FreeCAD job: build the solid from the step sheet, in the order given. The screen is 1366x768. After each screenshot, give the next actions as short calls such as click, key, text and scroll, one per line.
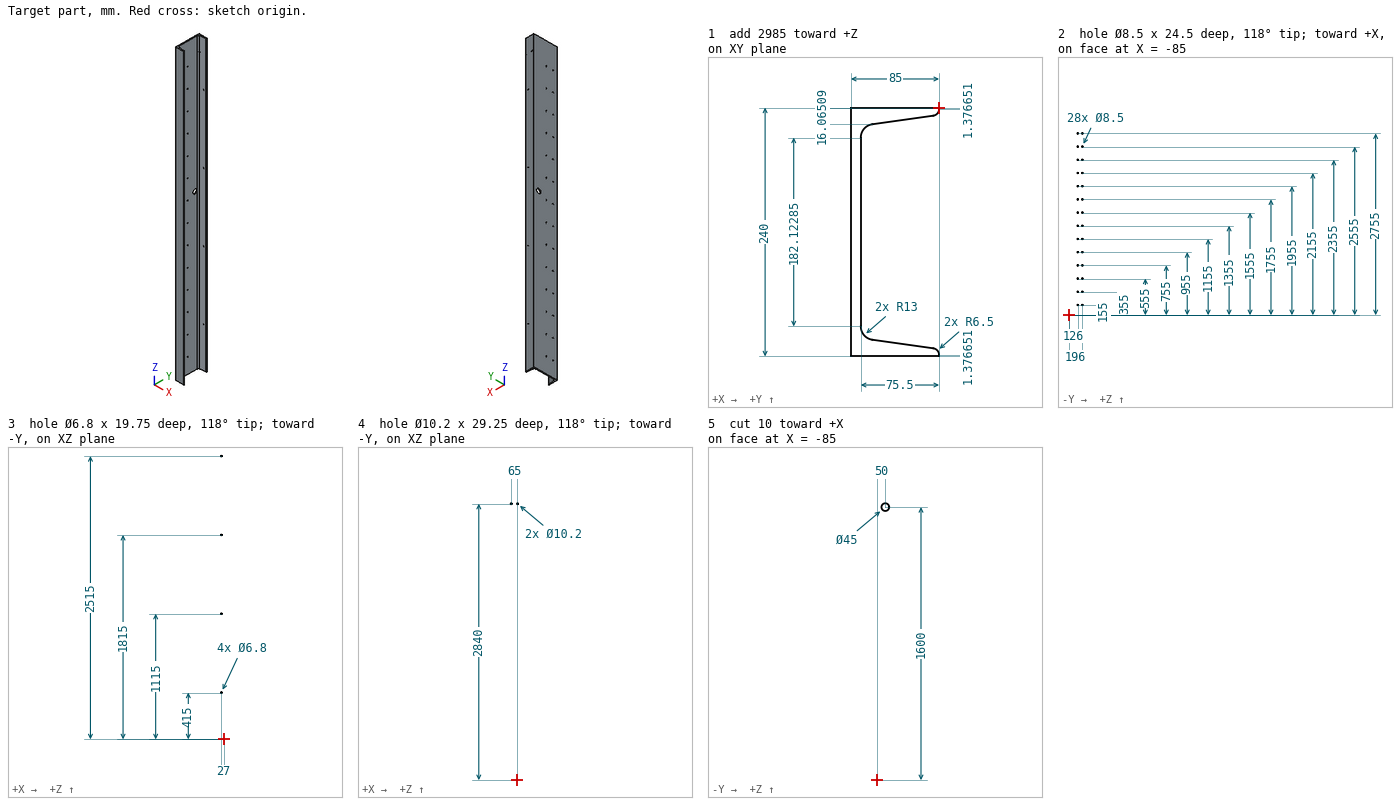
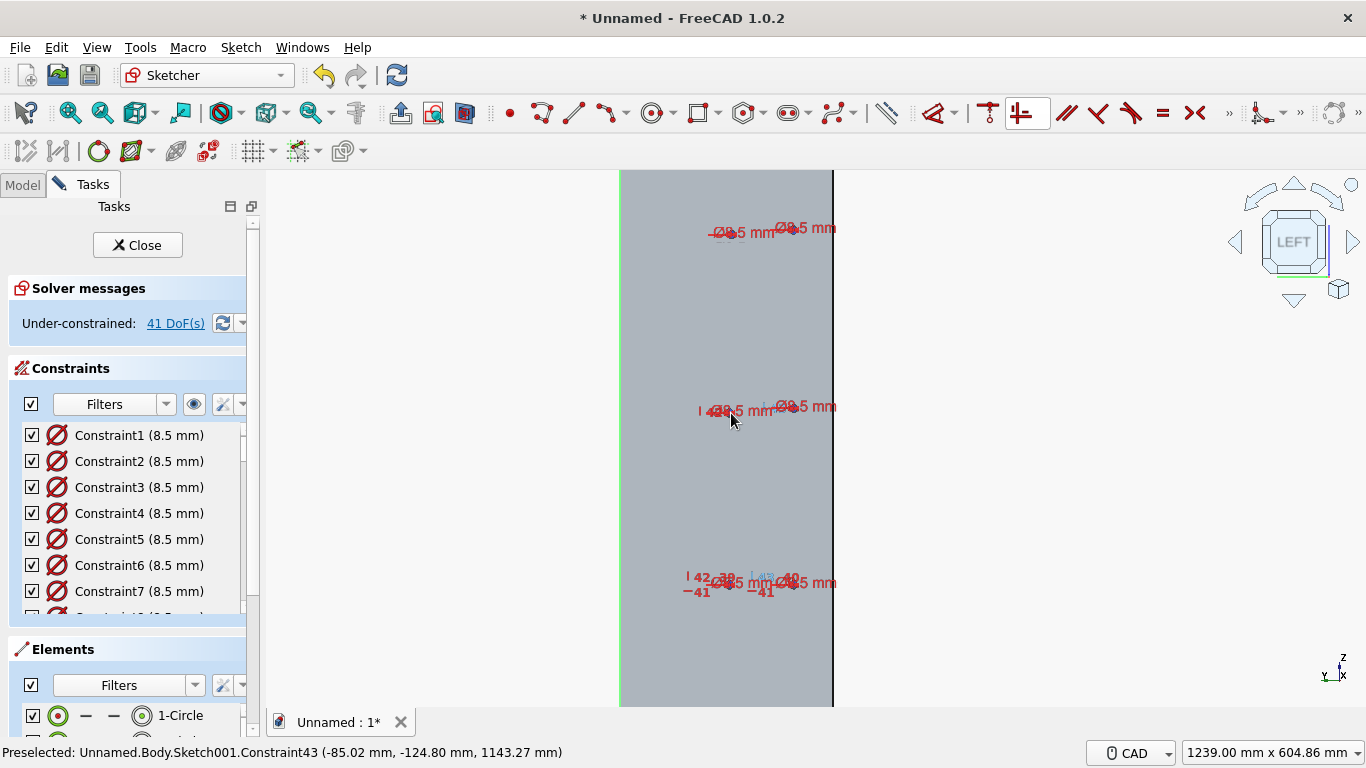
click(729, 413)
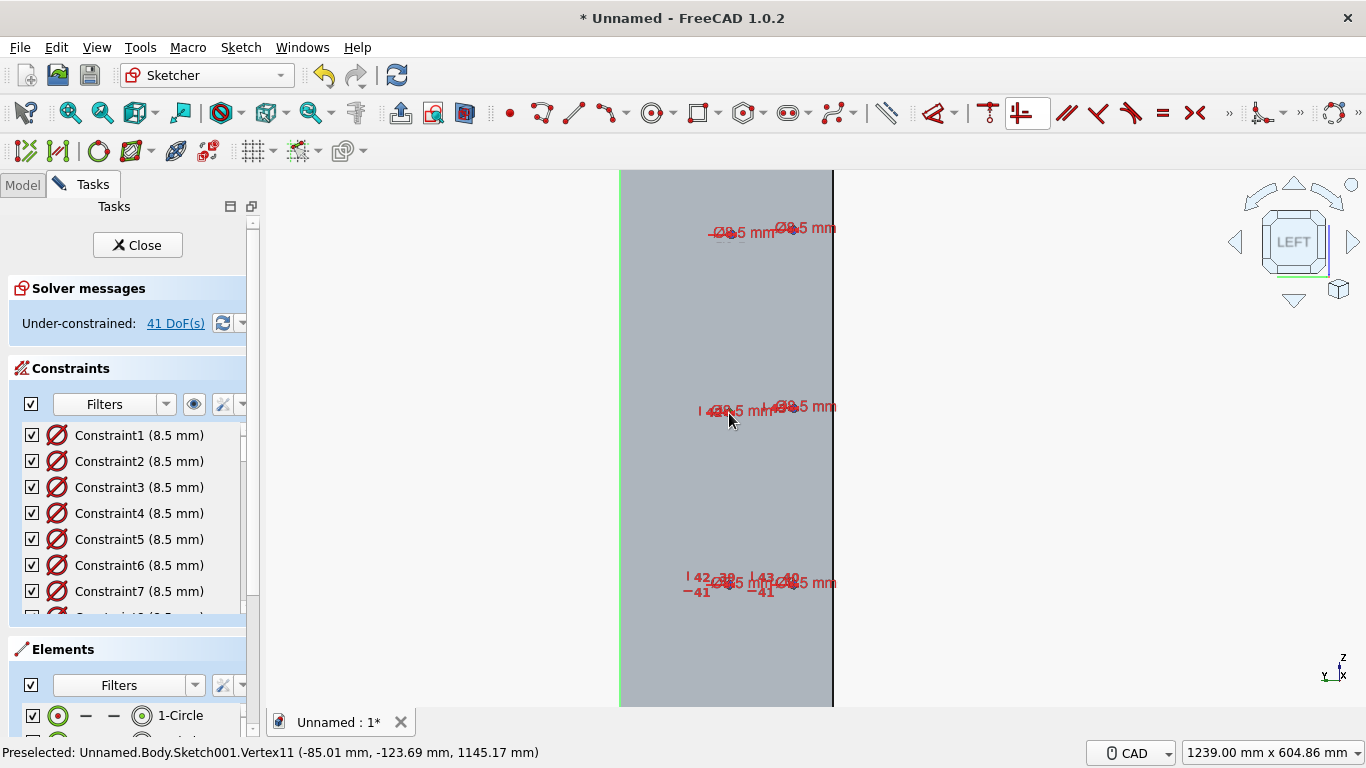
scroll(754, 475, down, 10)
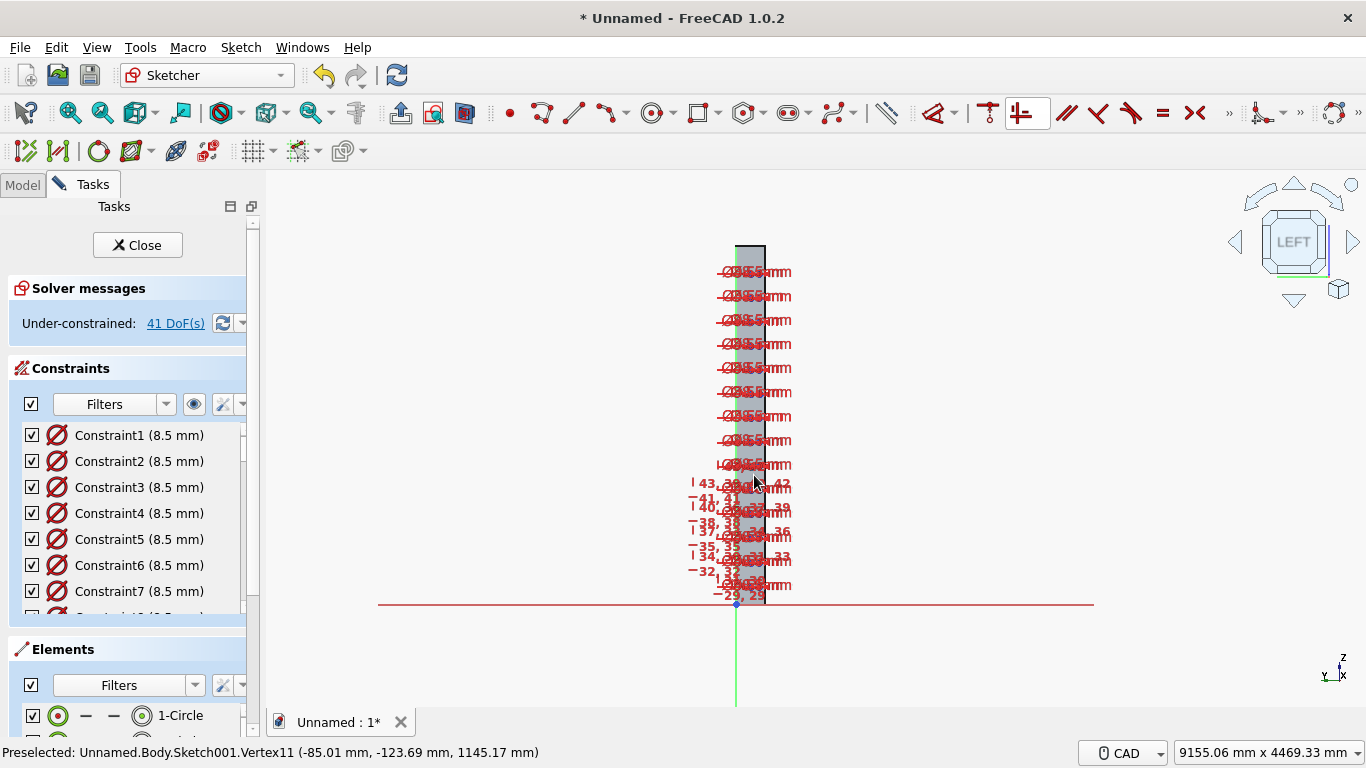
scroll(760, 466, up, 2)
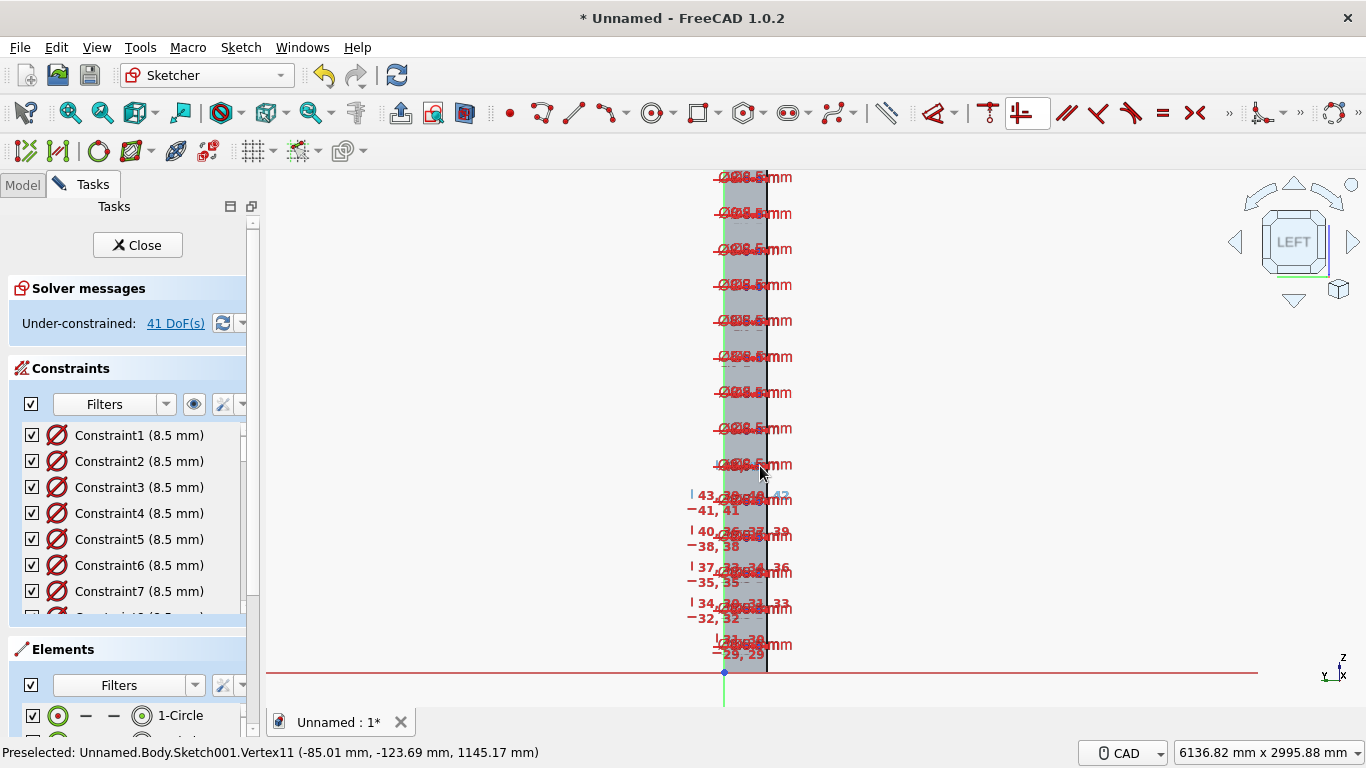
scroll(759, 466, up, 4)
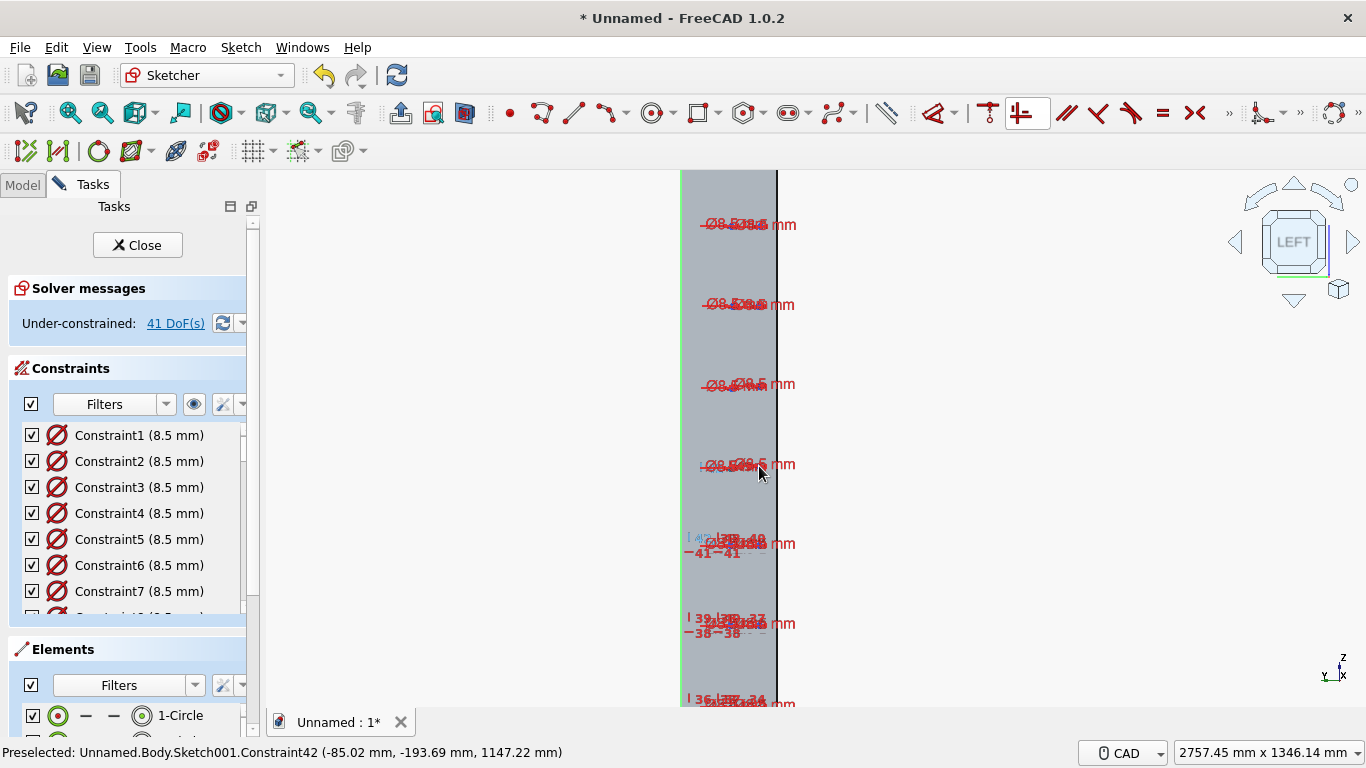
click(759, 466)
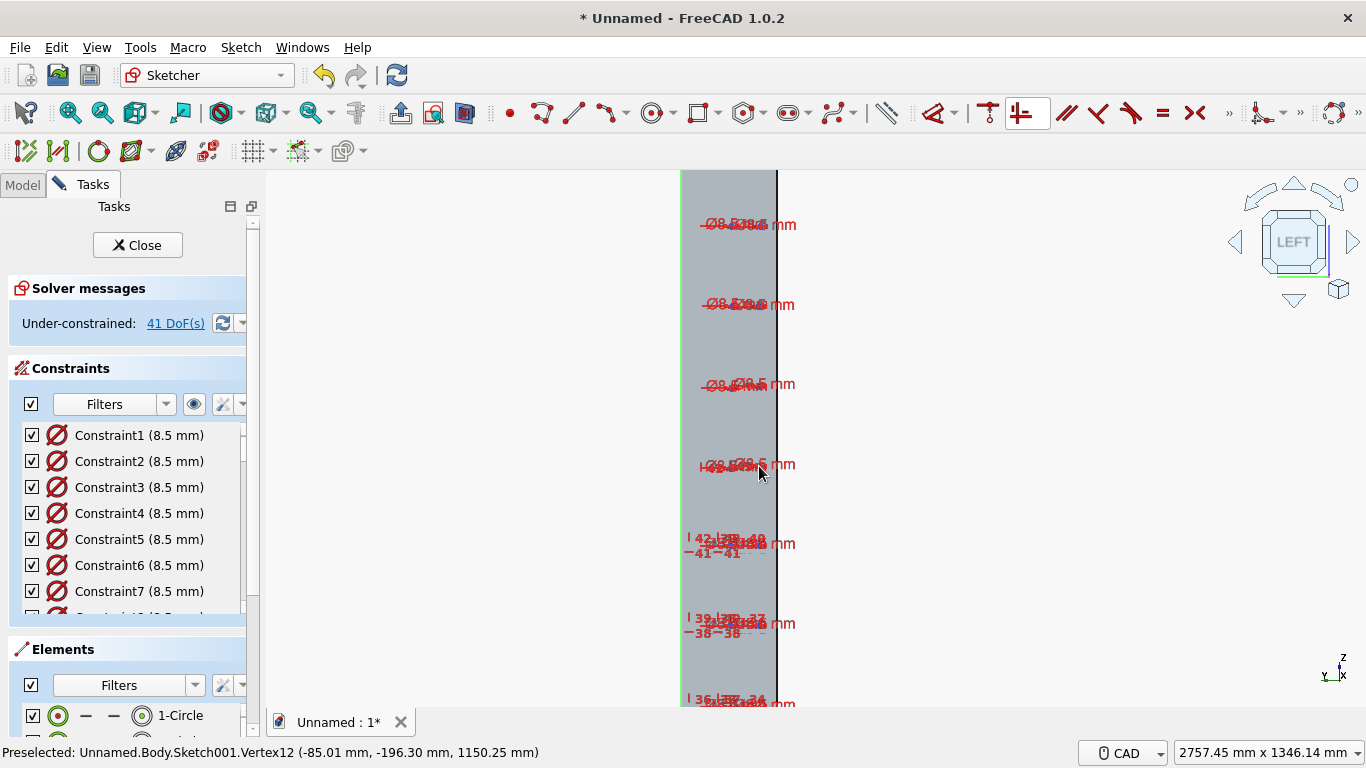
click(1044, 114)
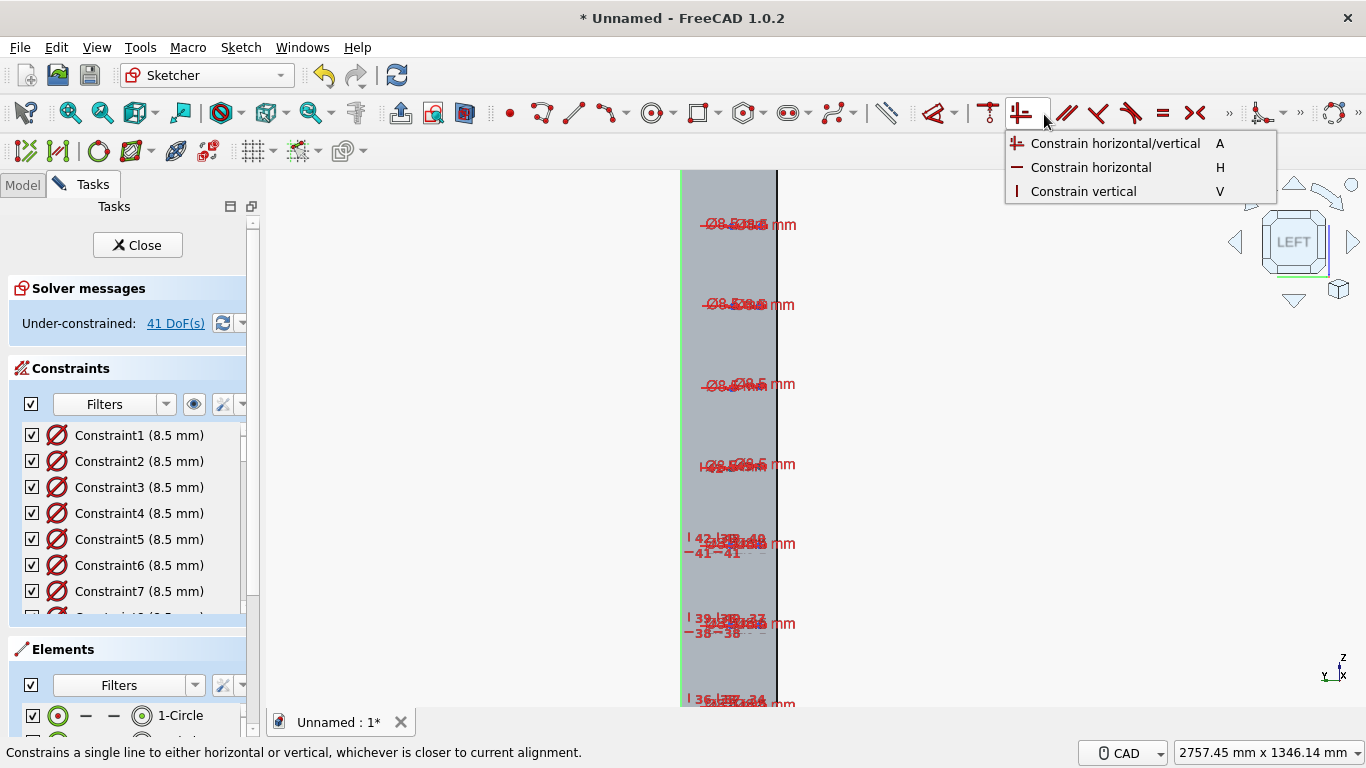
click(1141, 167)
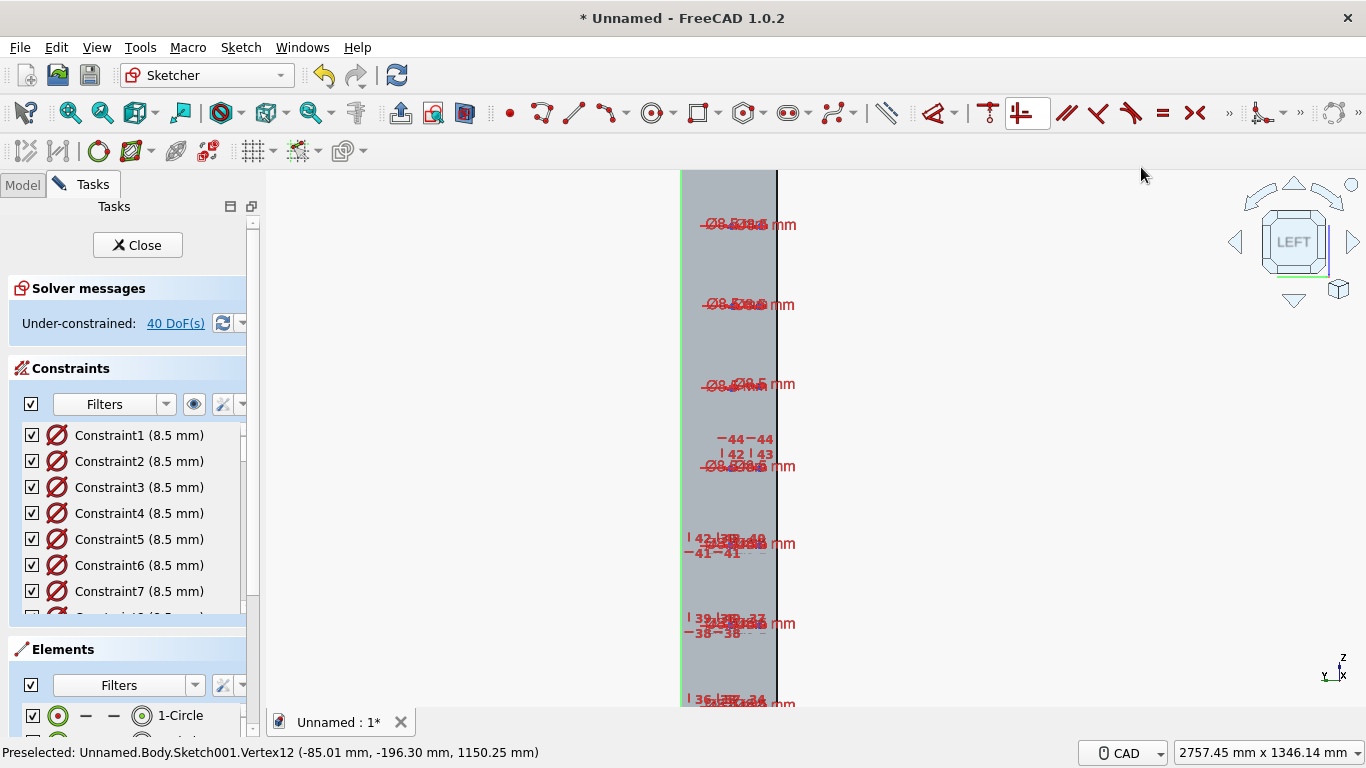
click(731, 468)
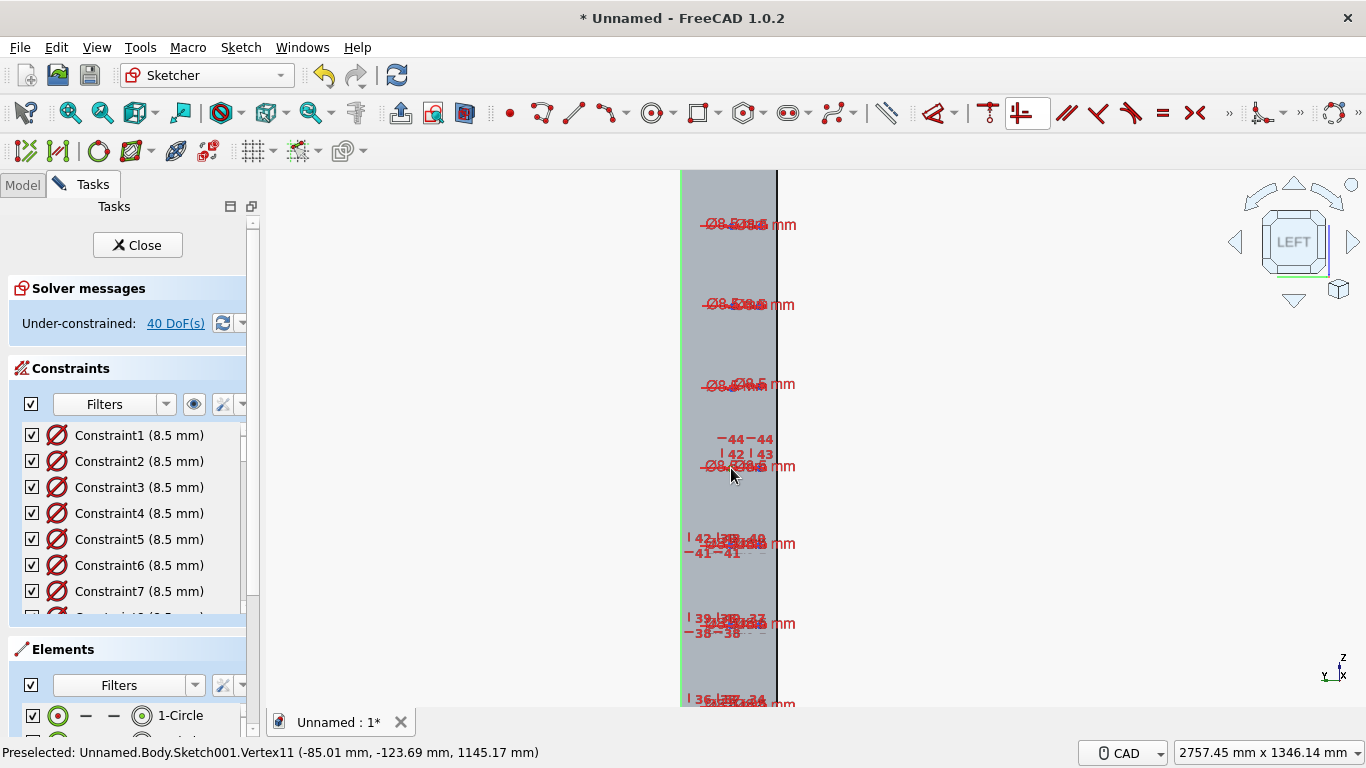
click(732, 388)